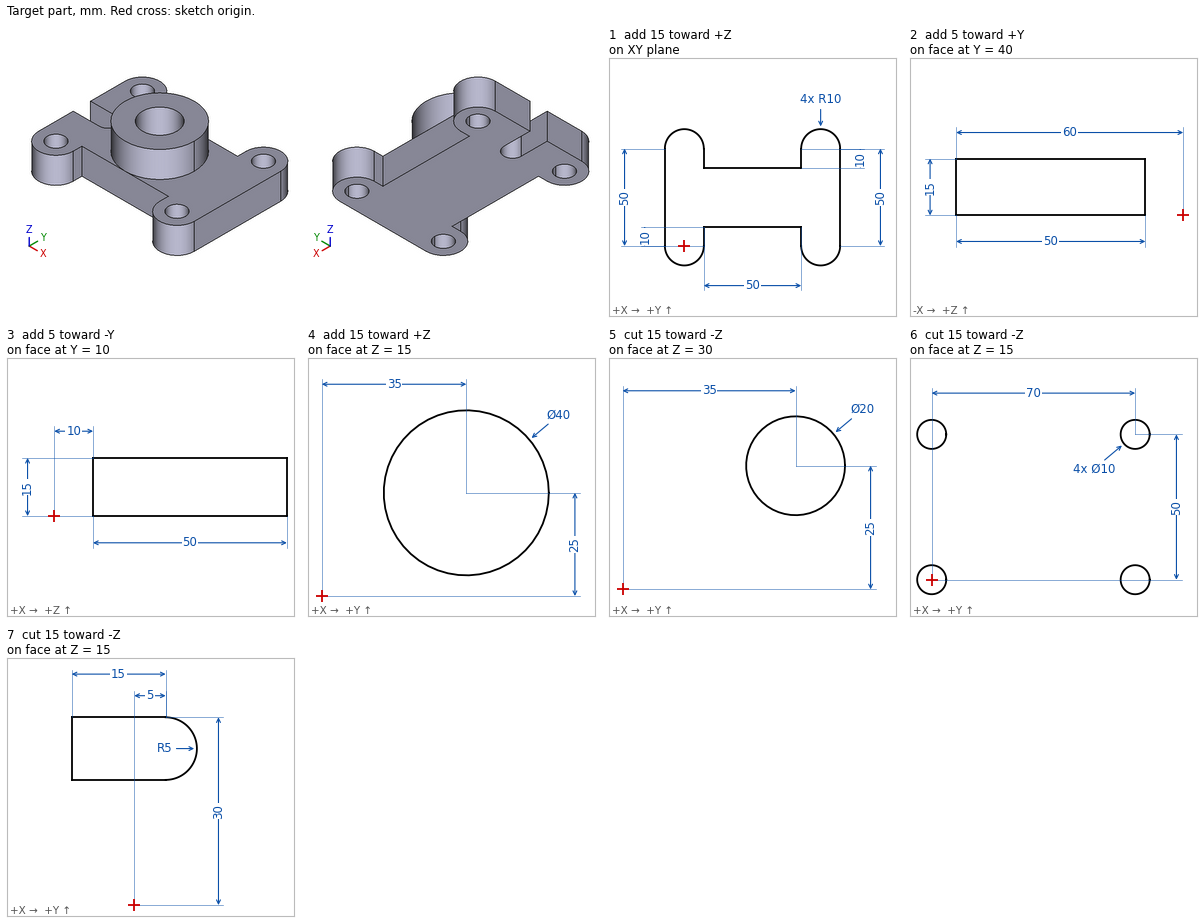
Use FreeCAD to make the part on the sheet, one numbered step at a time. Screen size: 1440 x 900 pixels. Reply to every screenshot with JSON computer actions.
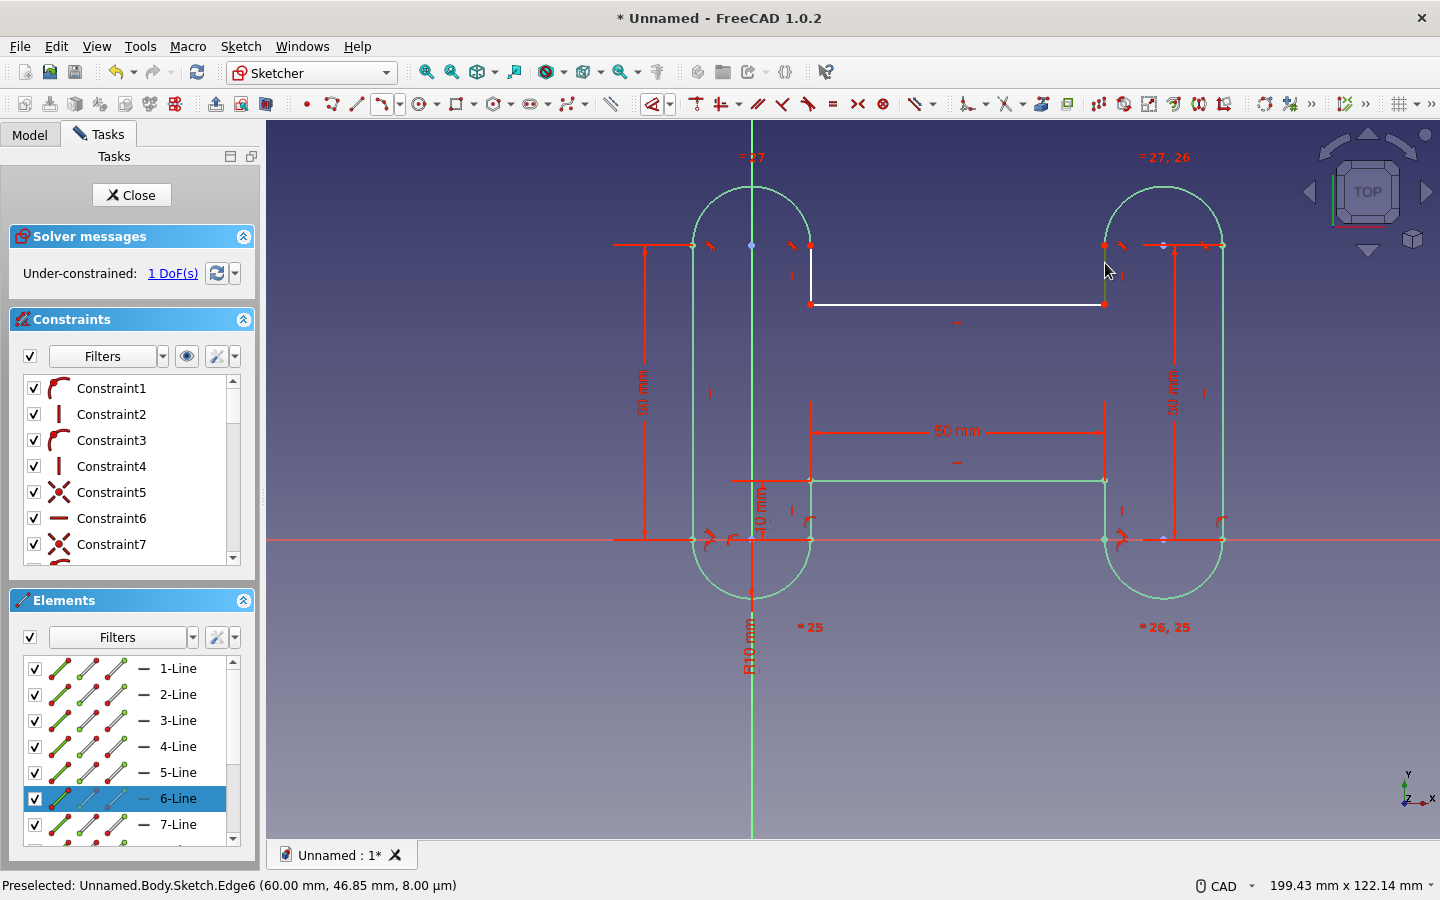
{"action": "left_click", "coordinate": [670, 104]}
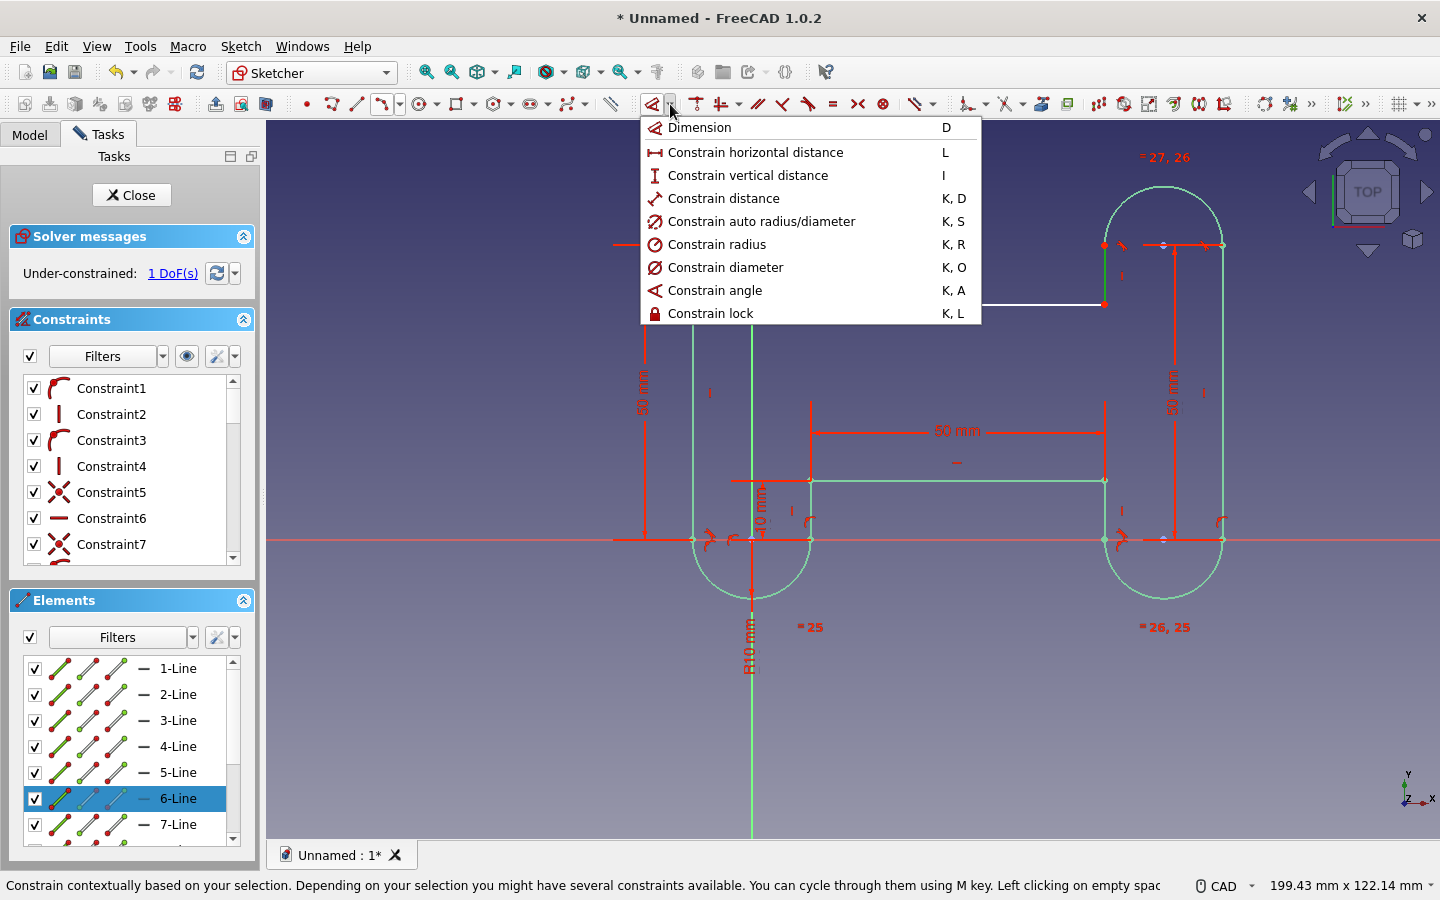
{"action": "left_click", "coordinate": [811, 176]}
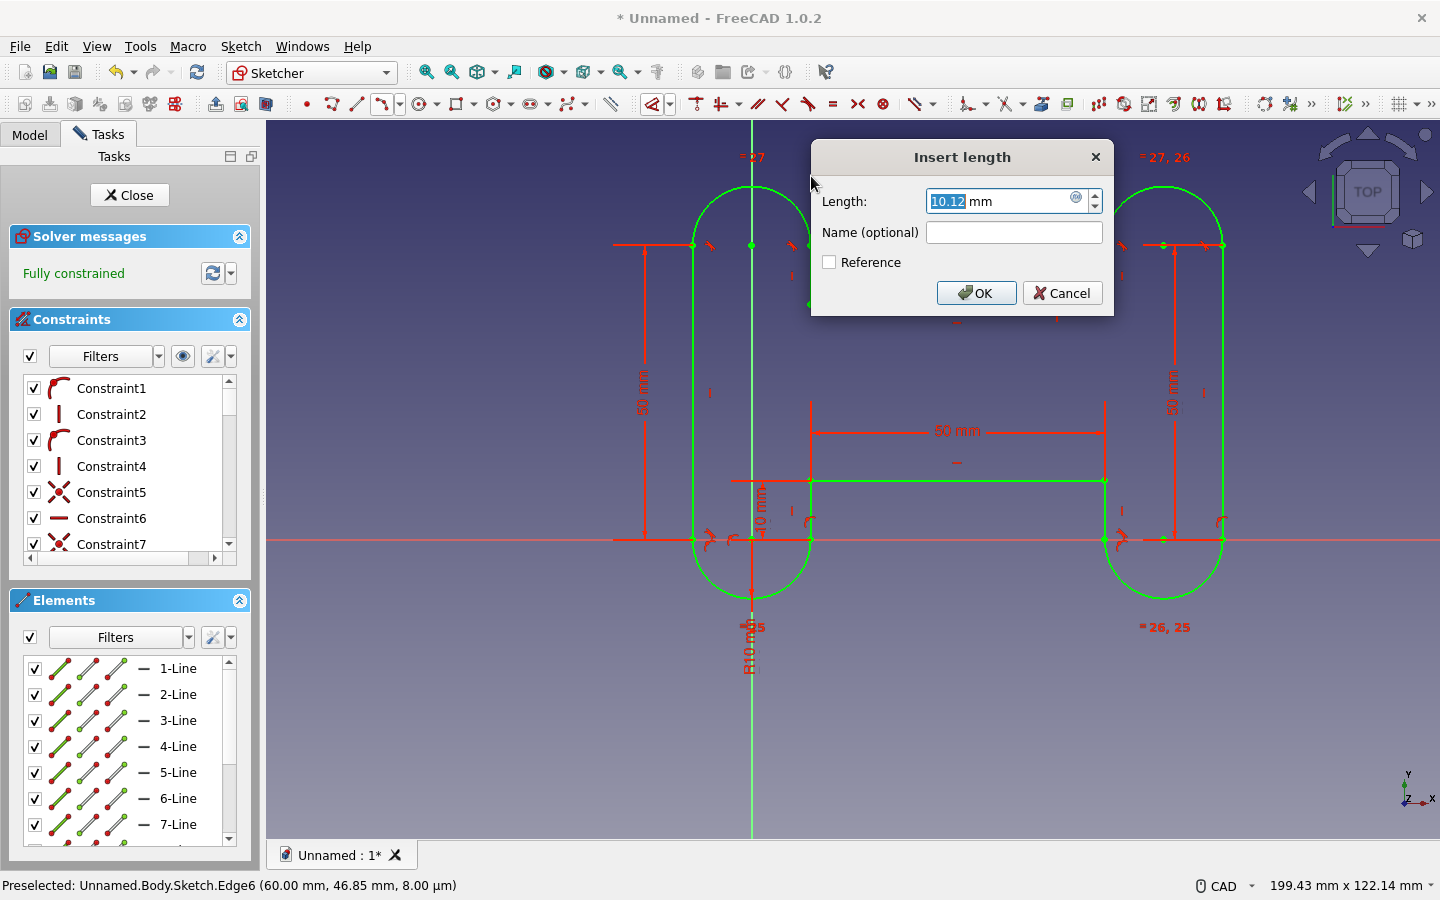
{"action": "type", "text": "10"}
{"action": "key", "text": "Return"}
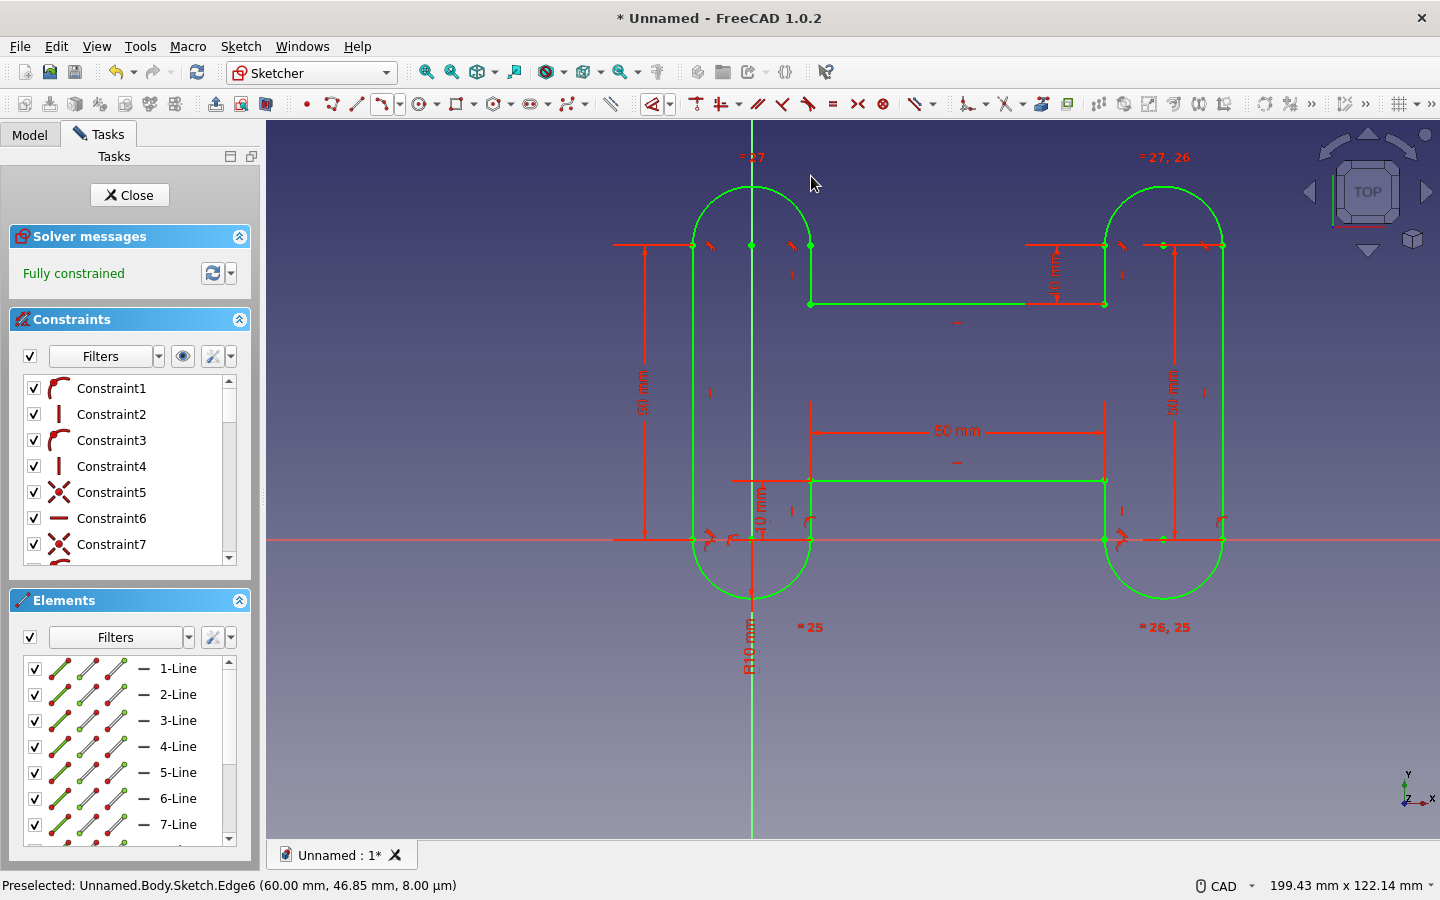
{"action": "left_click", "coordinate": [130, 195]}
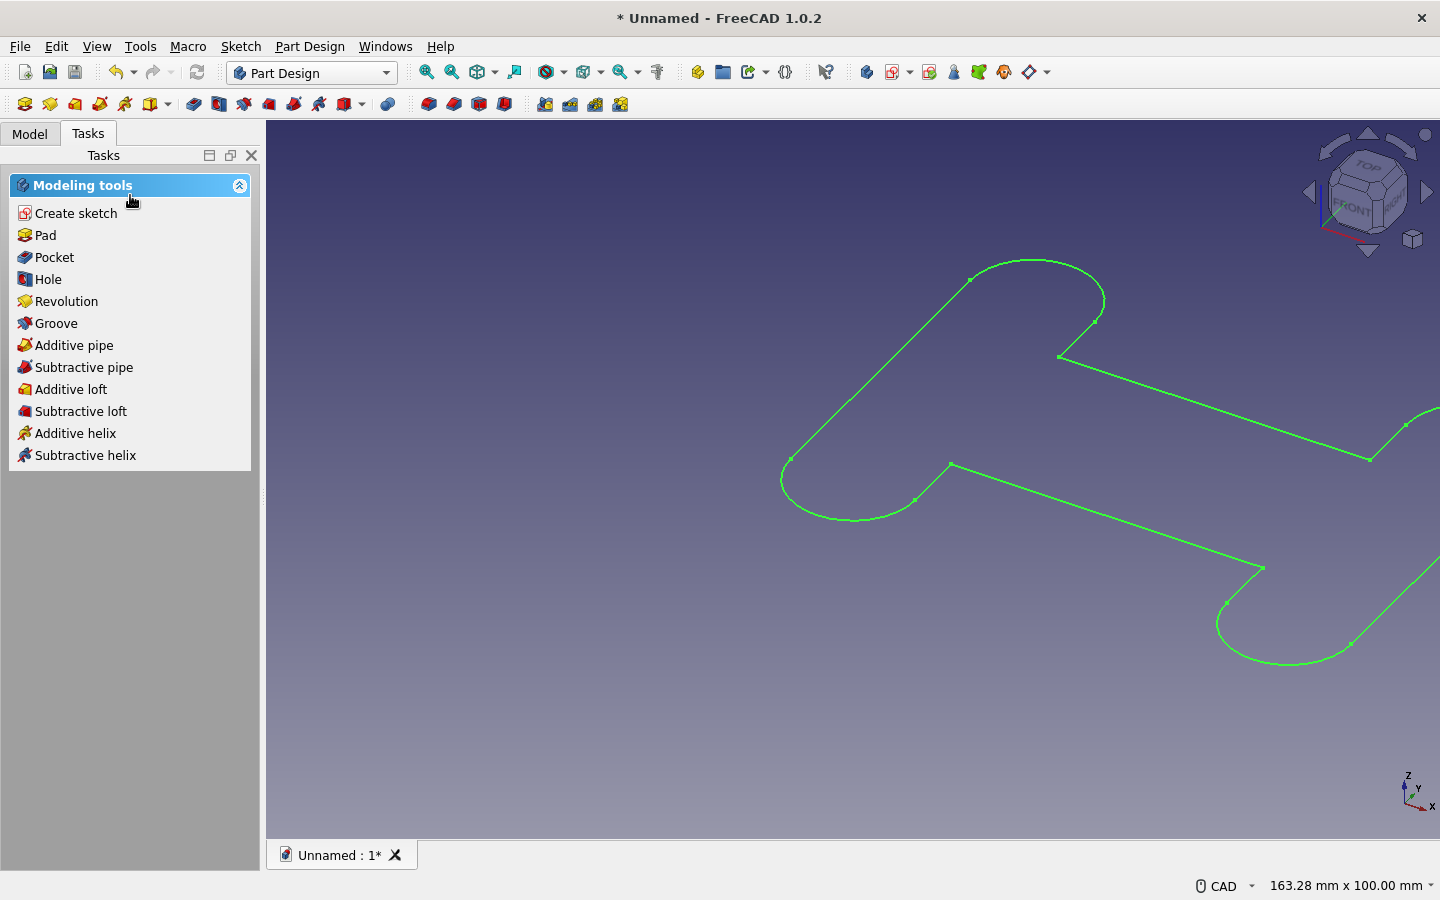
{"action": "left_click", "coordinate": [25, 104]}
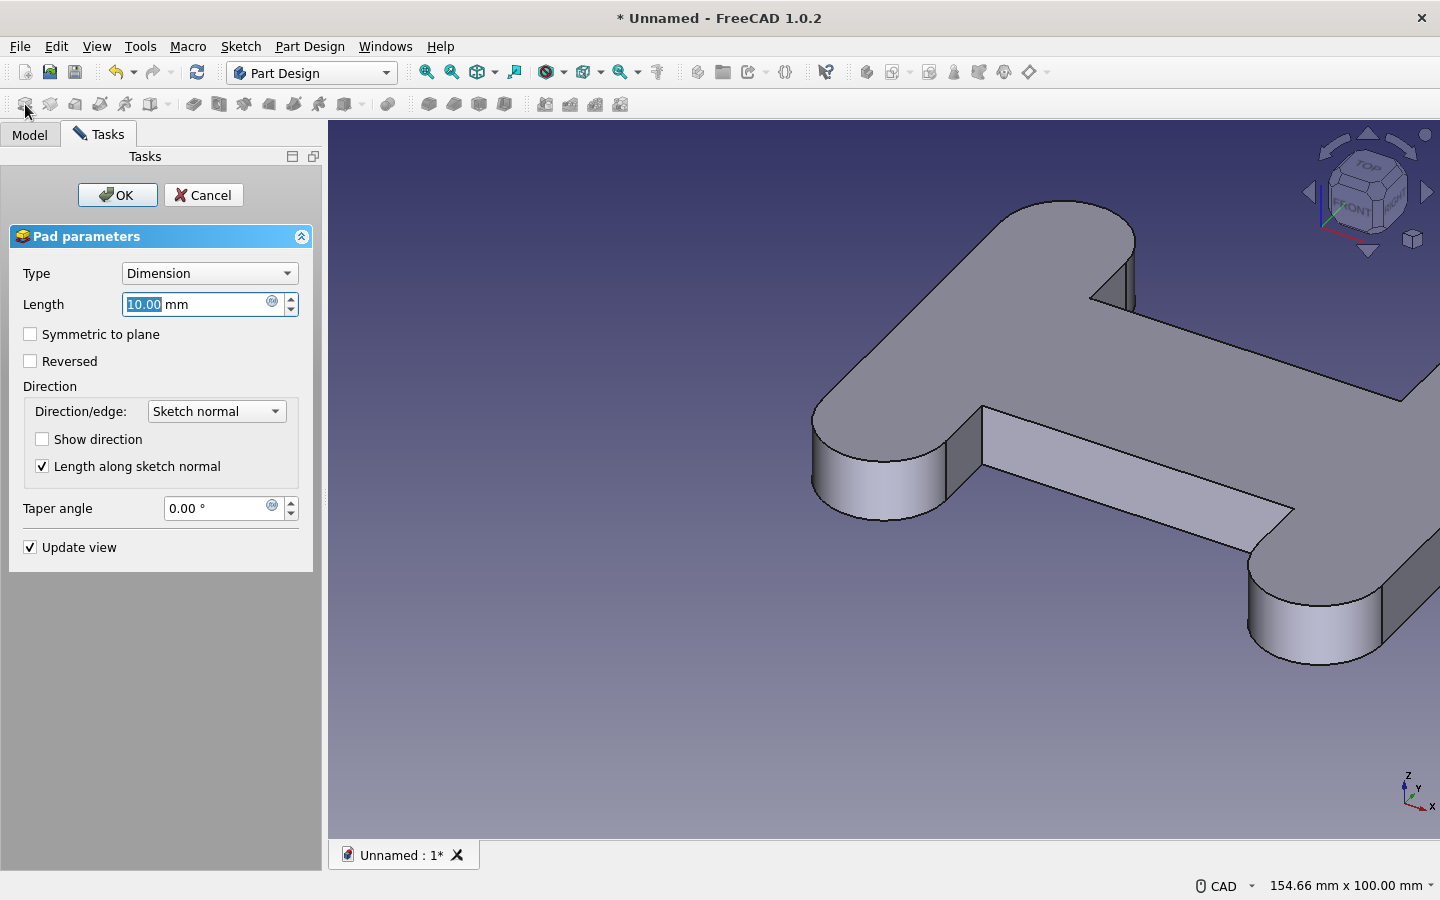
{"action": "type", "text": "15"}
{"action": "key", "text": "Tab"}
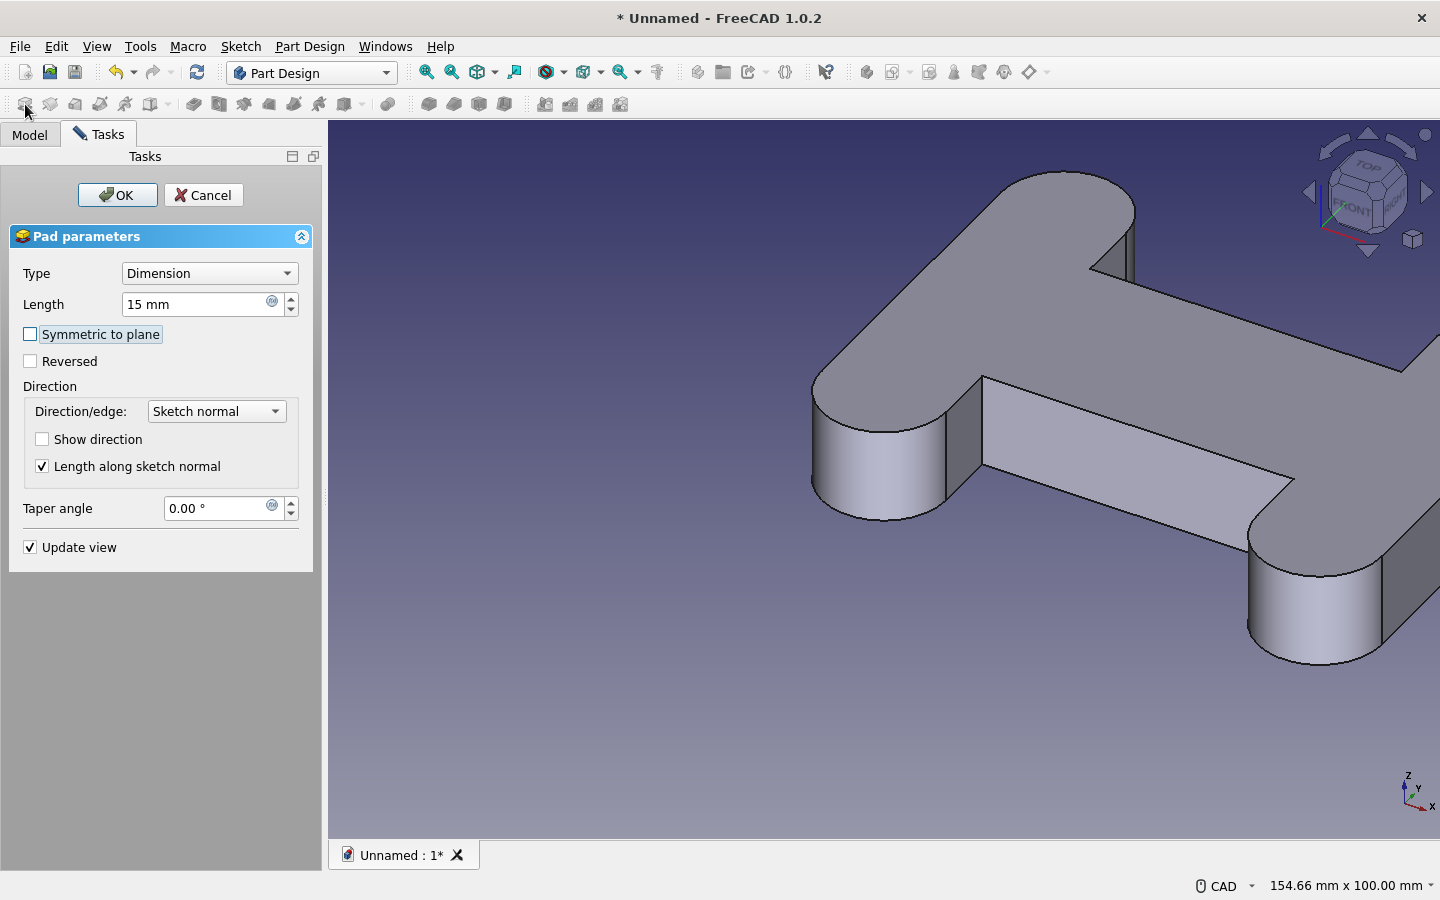
{"action": "left_click", "coordinate": [118, 195]}